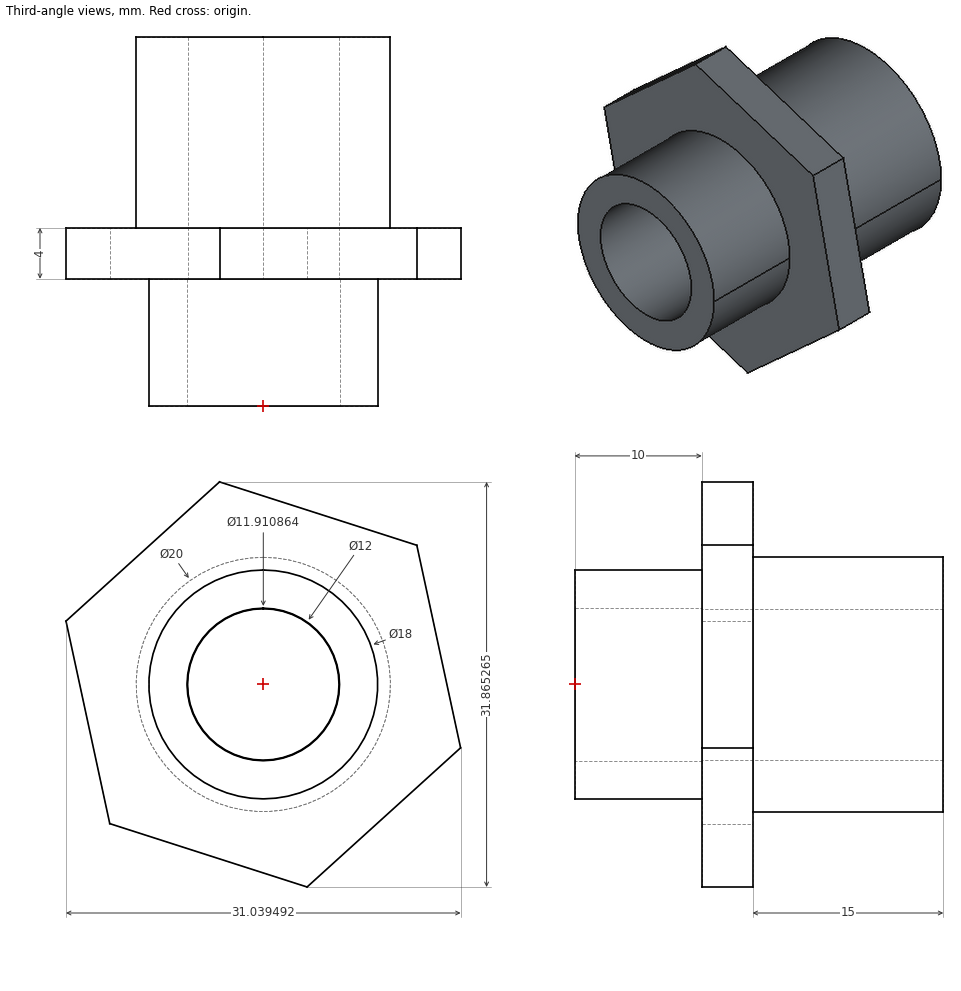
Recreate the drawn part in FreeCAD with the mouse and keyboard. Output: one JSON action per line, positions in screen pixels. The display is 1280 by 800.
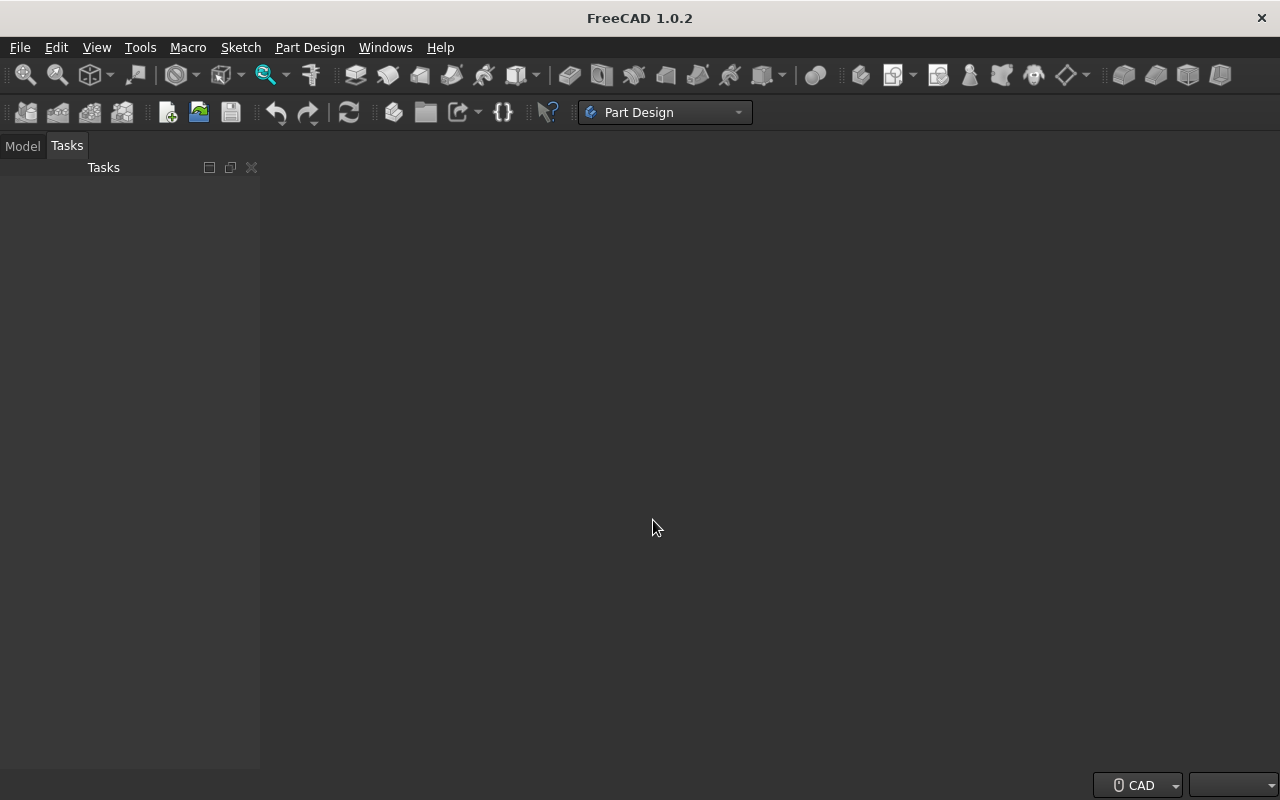
{"action": "left_click", "coordinate": [168, 112]}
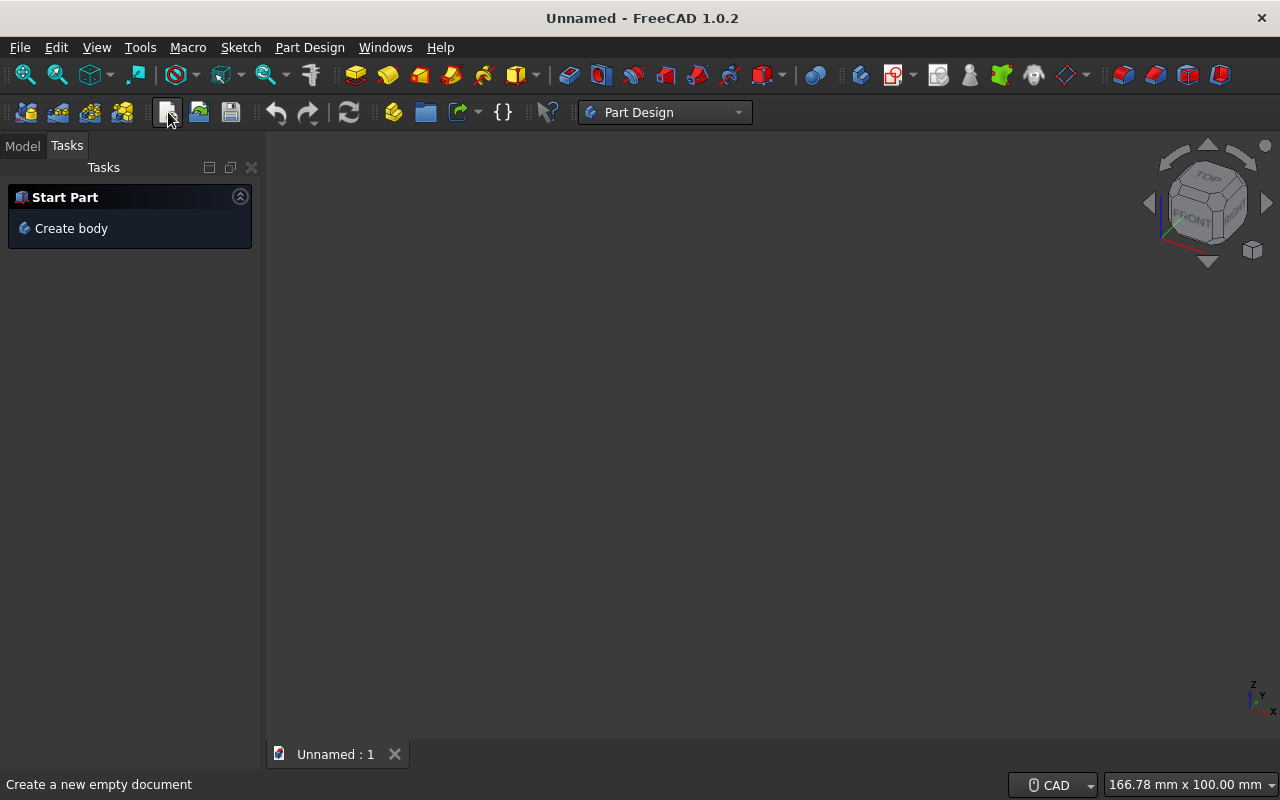
{"action": "left_click", "coordinate": [894, 76]}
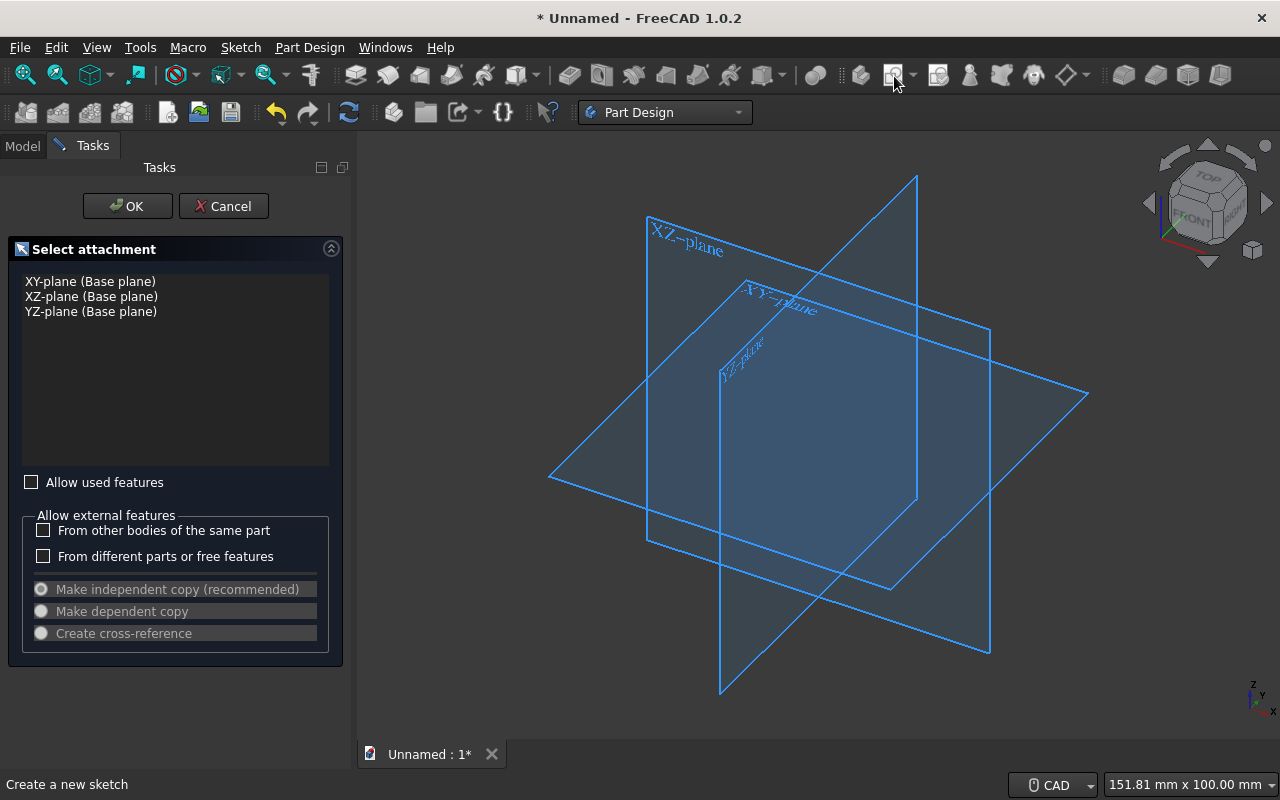
{"action": "left_click", "coordinate": [82, 296]}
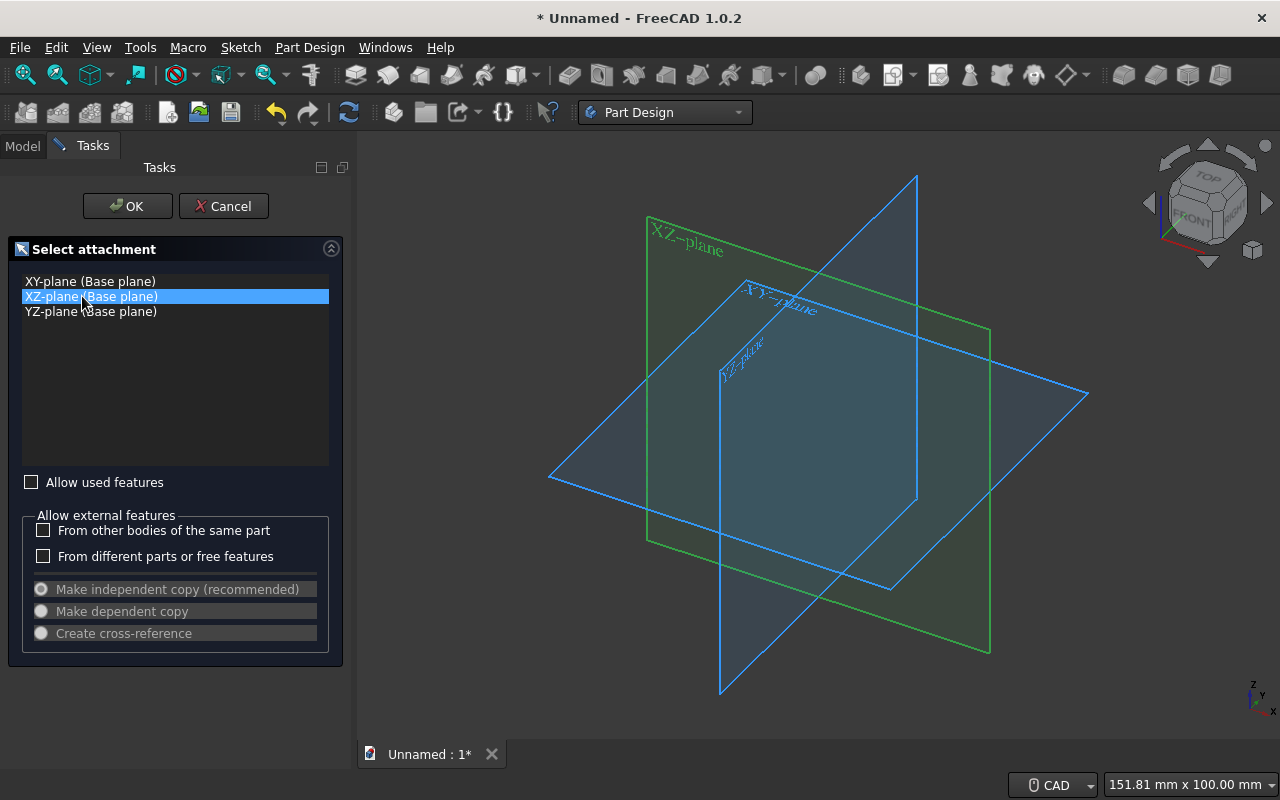
{"action": "left_click", "coordinate": [128, 206]}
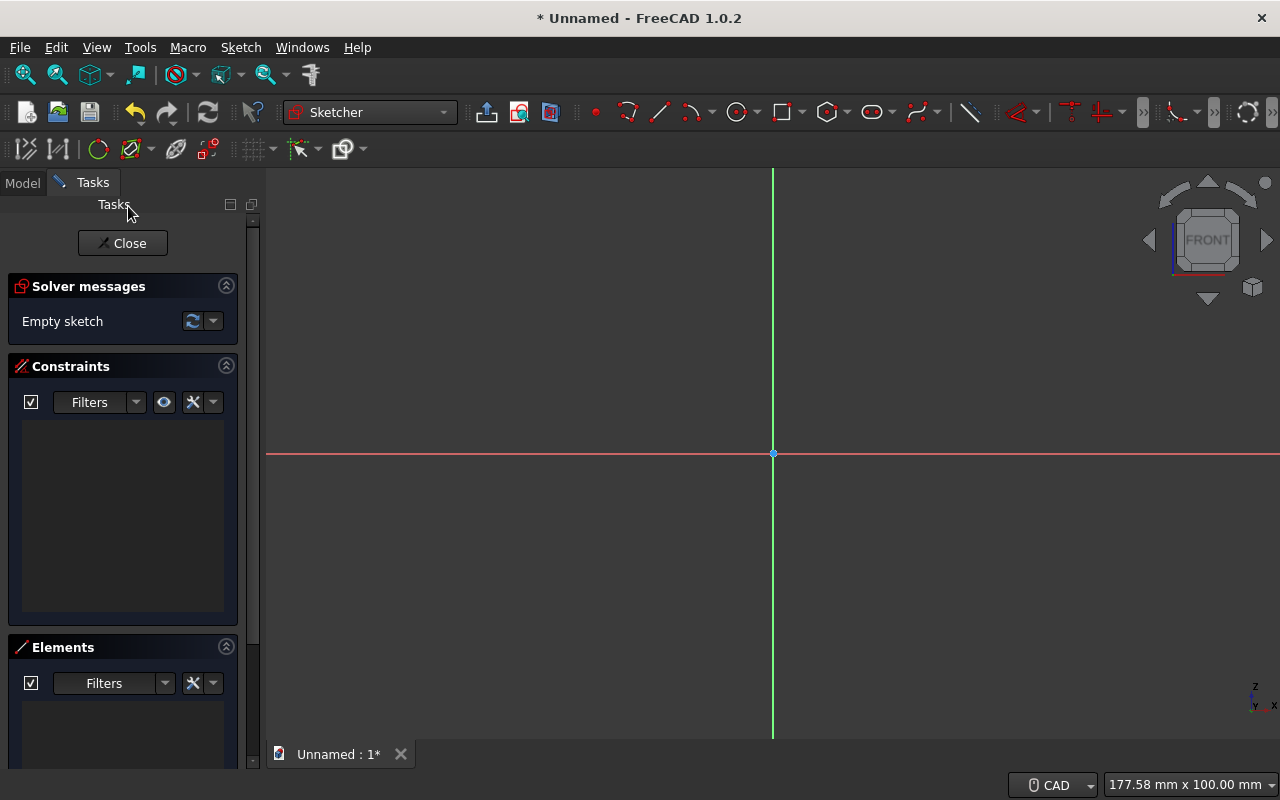
{"action": "scroll", "coordinate": [803, 454], "scroll_direction": "up", "scroll_amount": 6}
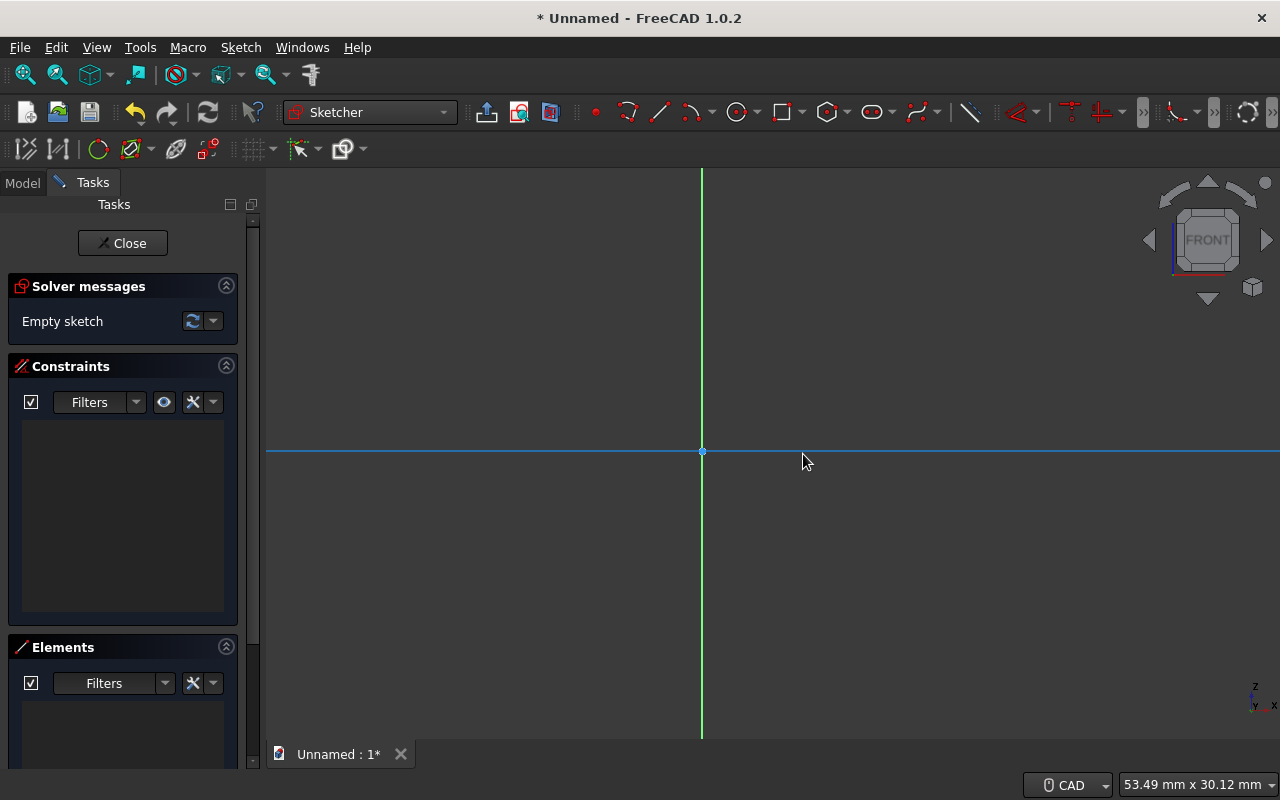
{"action": "left_click", "coordinate": [738, 112]}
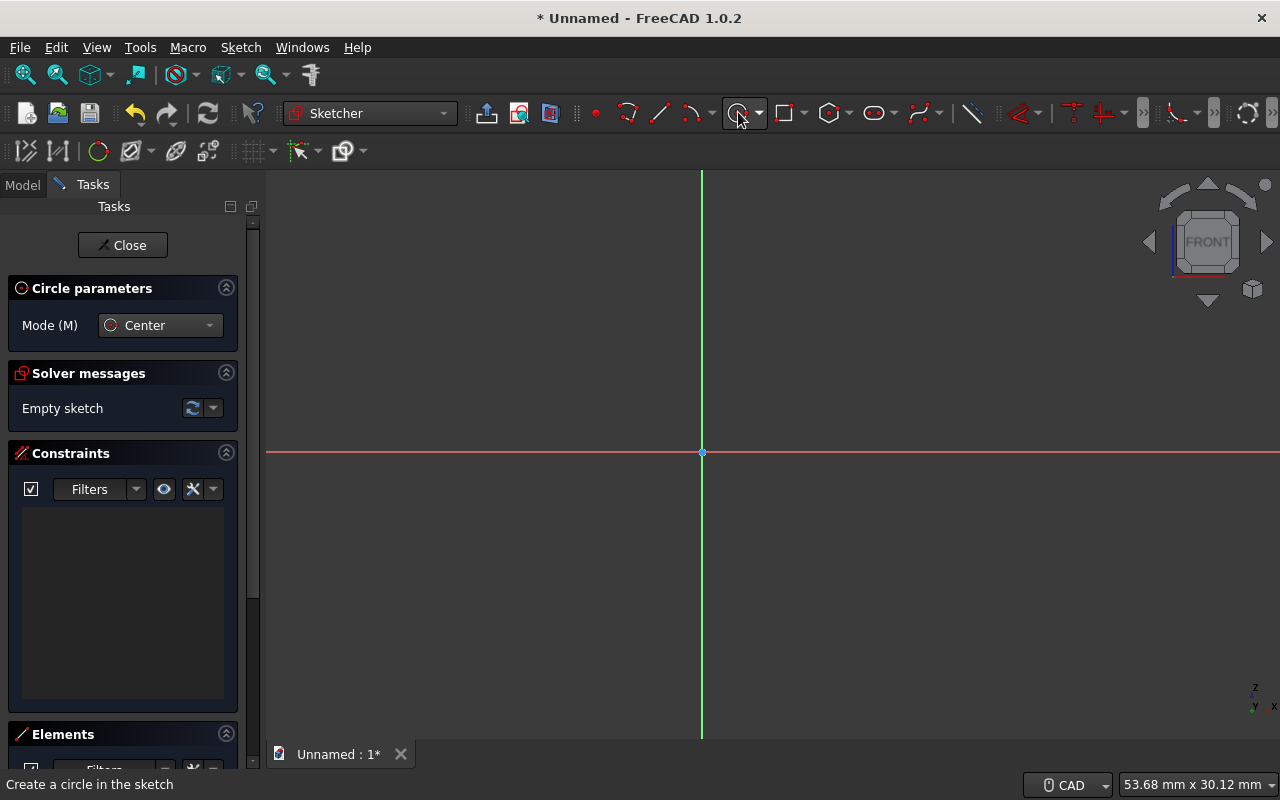
{"action": "left_click", "coordinate": [702, 452]}
{"action": "mouse_move", "coordinate": [823, 332]}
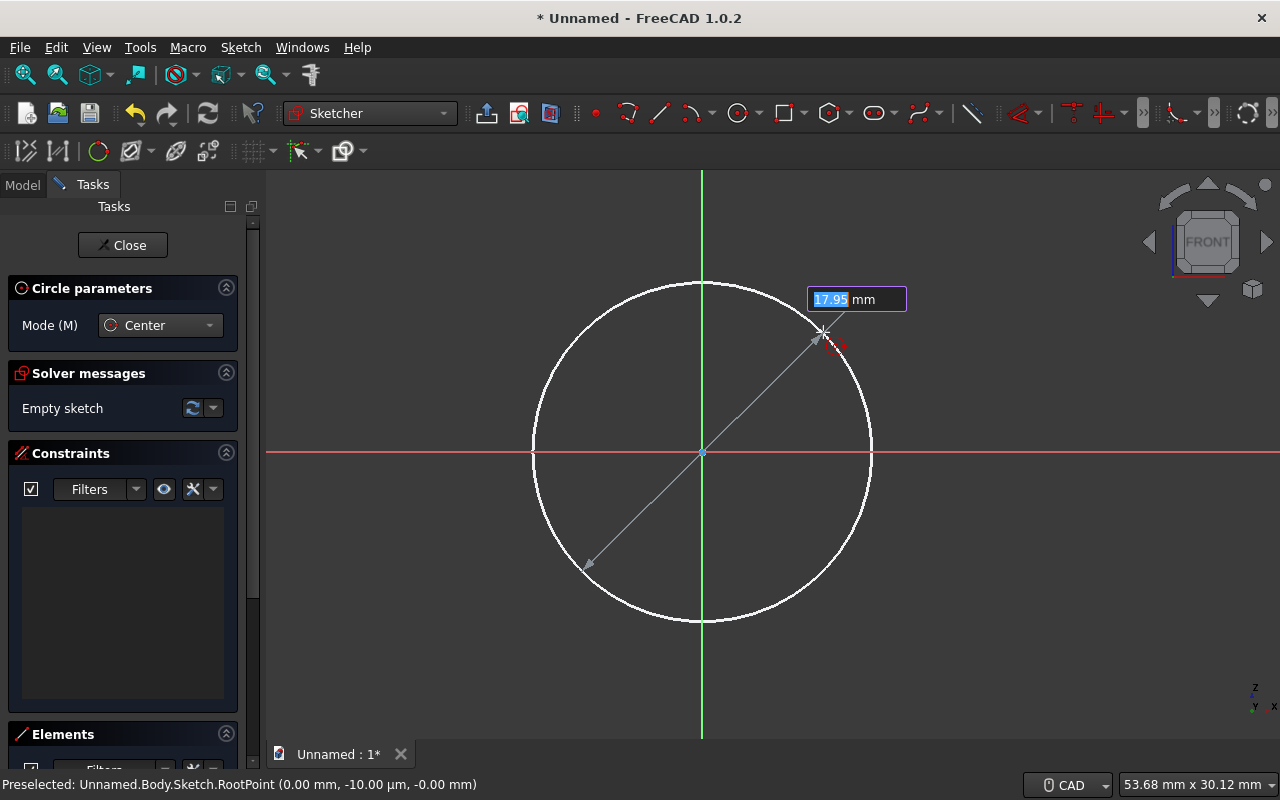
{"action": "type", "text": "18"}
{"action": "key", "text": "Return"}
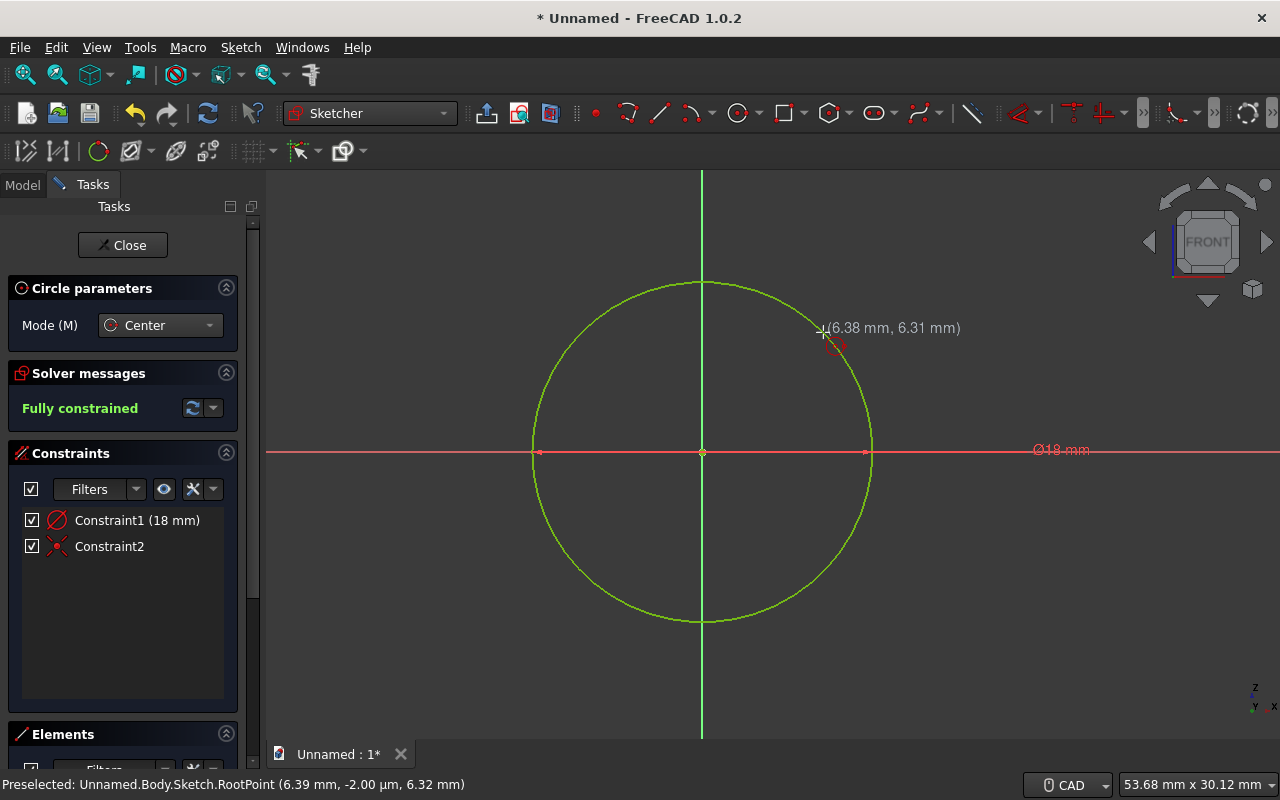
{"action": "left_click", "coordinate": [702, 452]}
{"action": "mouse_move", "coordinate": [783, 372]}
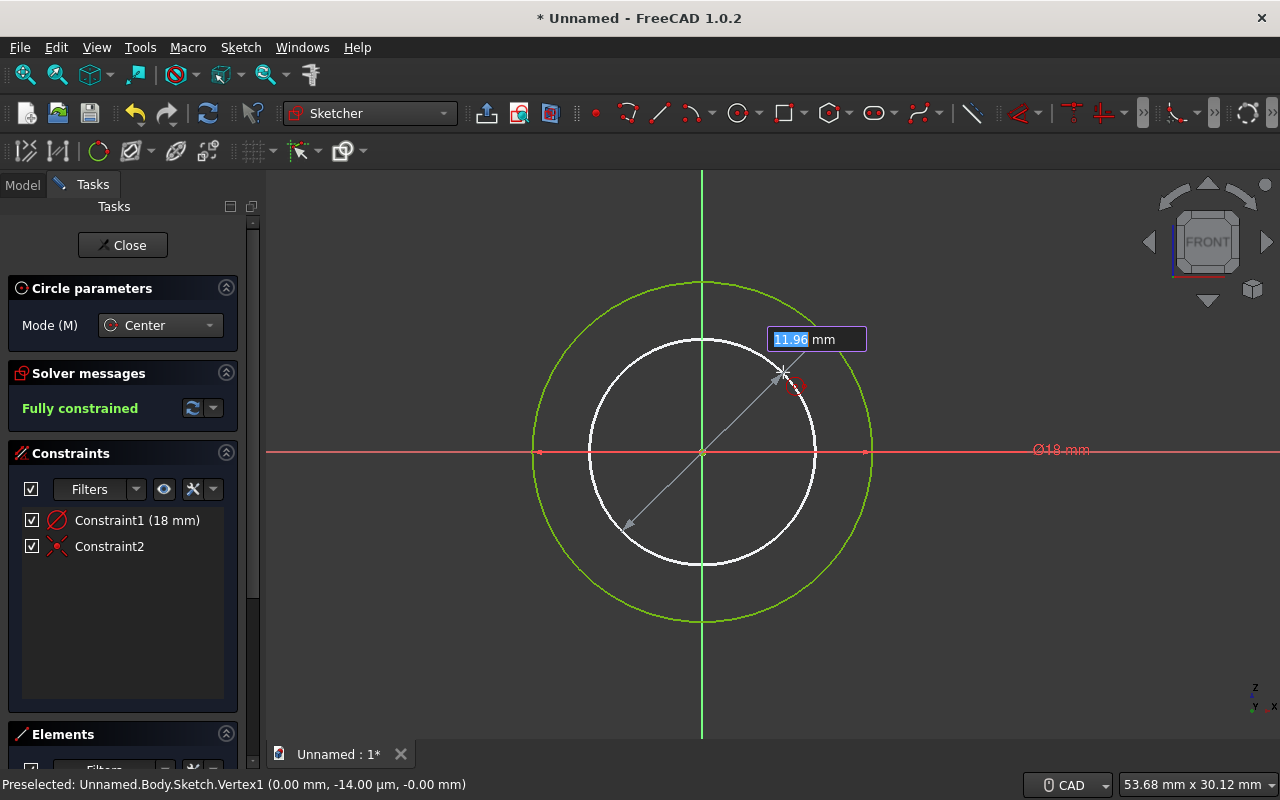
{"action": "type", "text": "12"}
{"action": "key", "text": "Return"}
{"action": "key", "text": "Escape"}